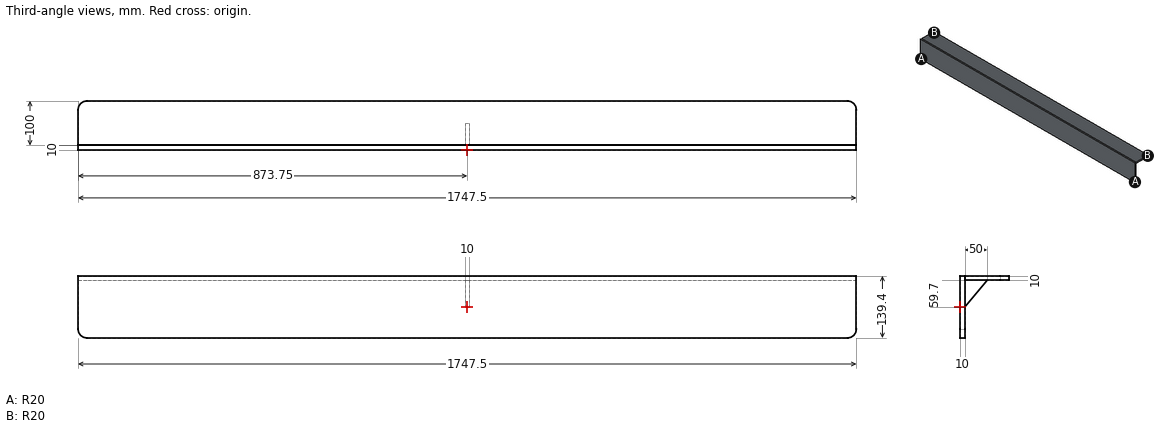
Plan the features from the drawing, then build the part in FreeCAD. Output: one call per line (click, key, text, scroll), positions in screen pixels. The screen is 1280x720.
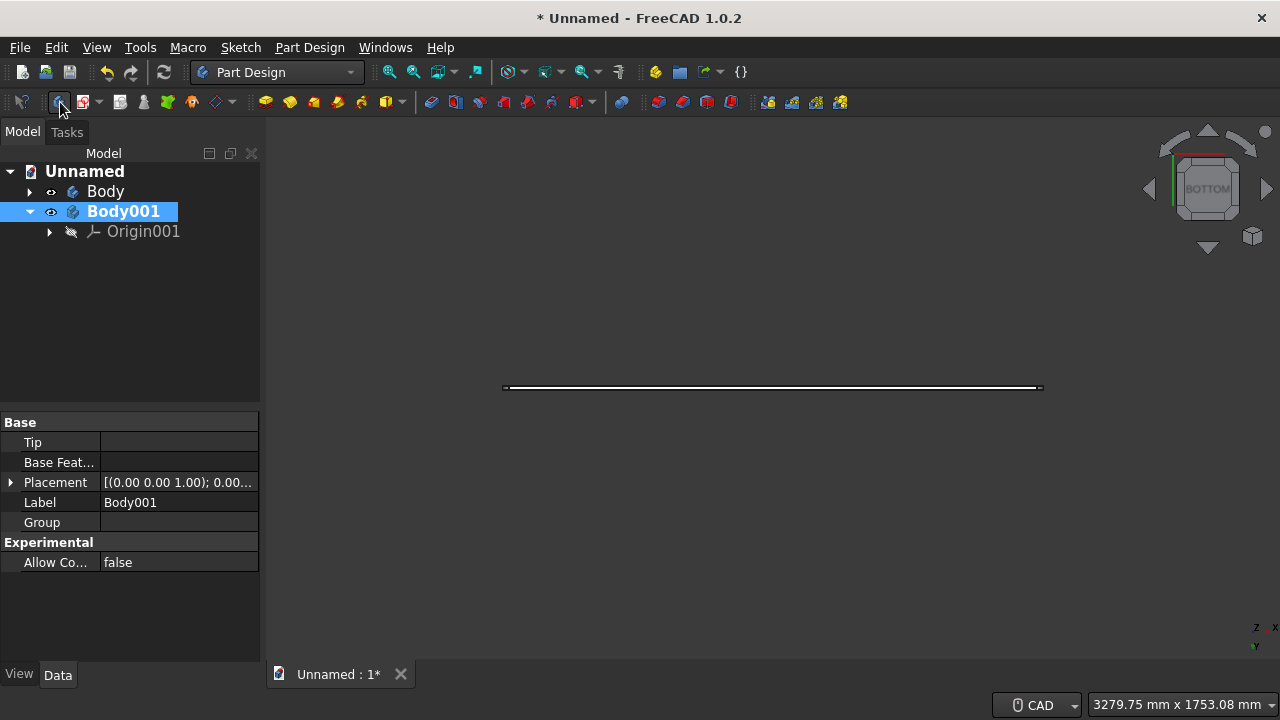
click(50, 232)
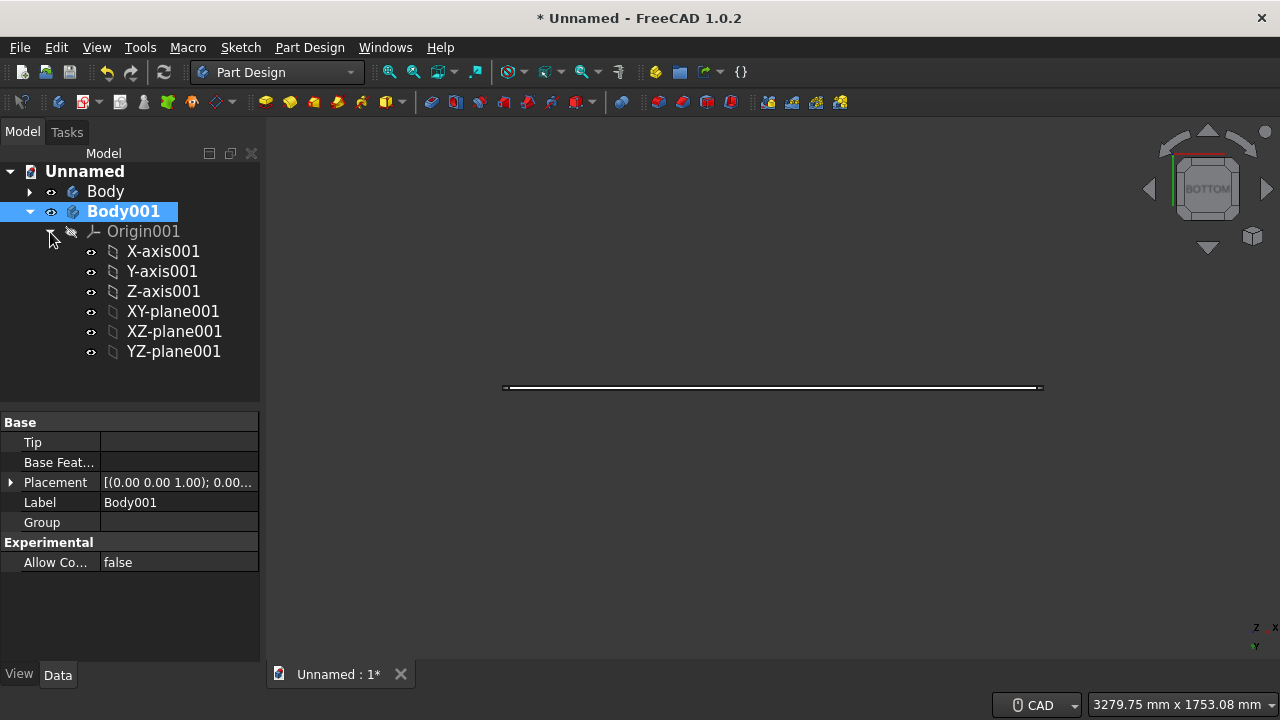
click(136, 312)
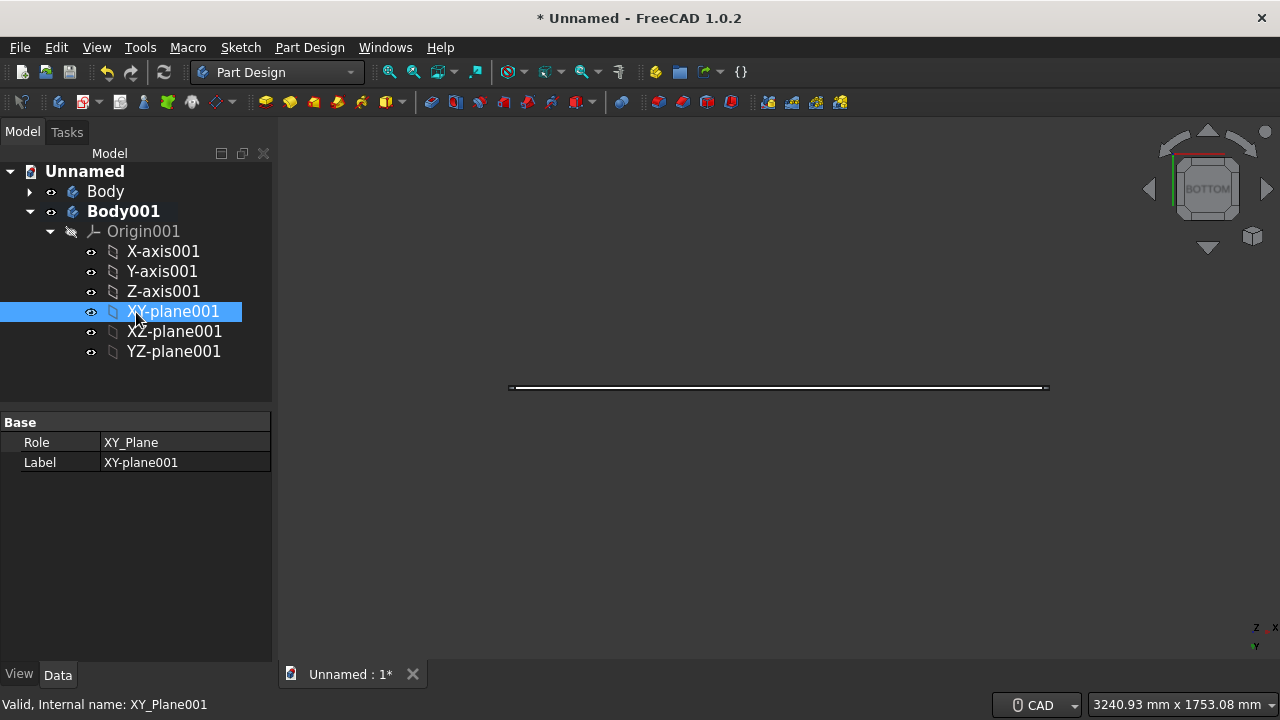
click(216, 102)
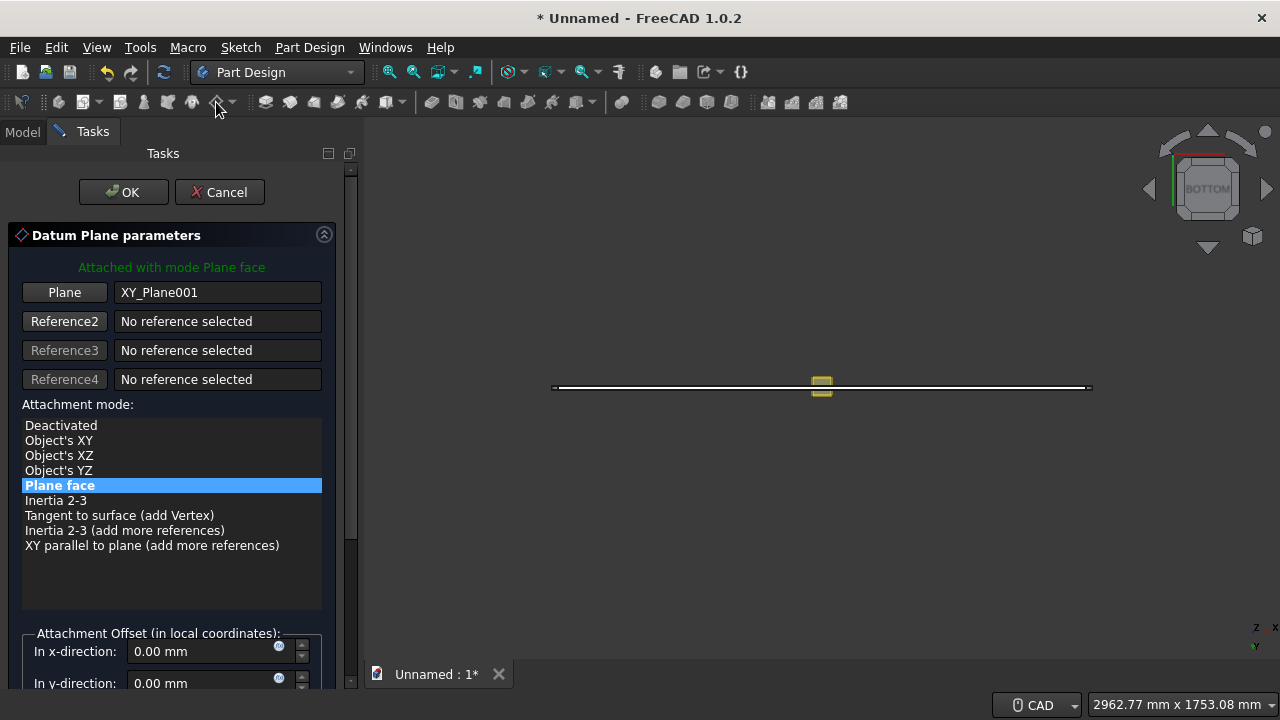
scroll(351, 426, down, 2)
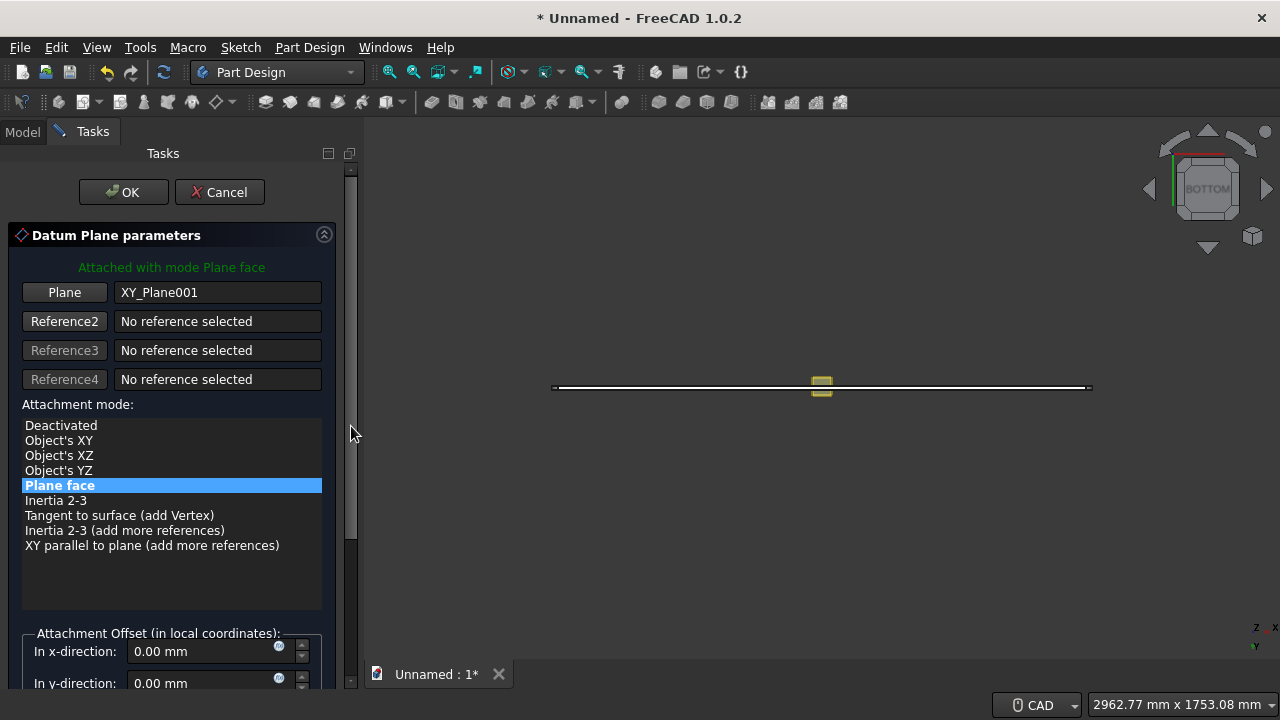
triple_click(210, 595)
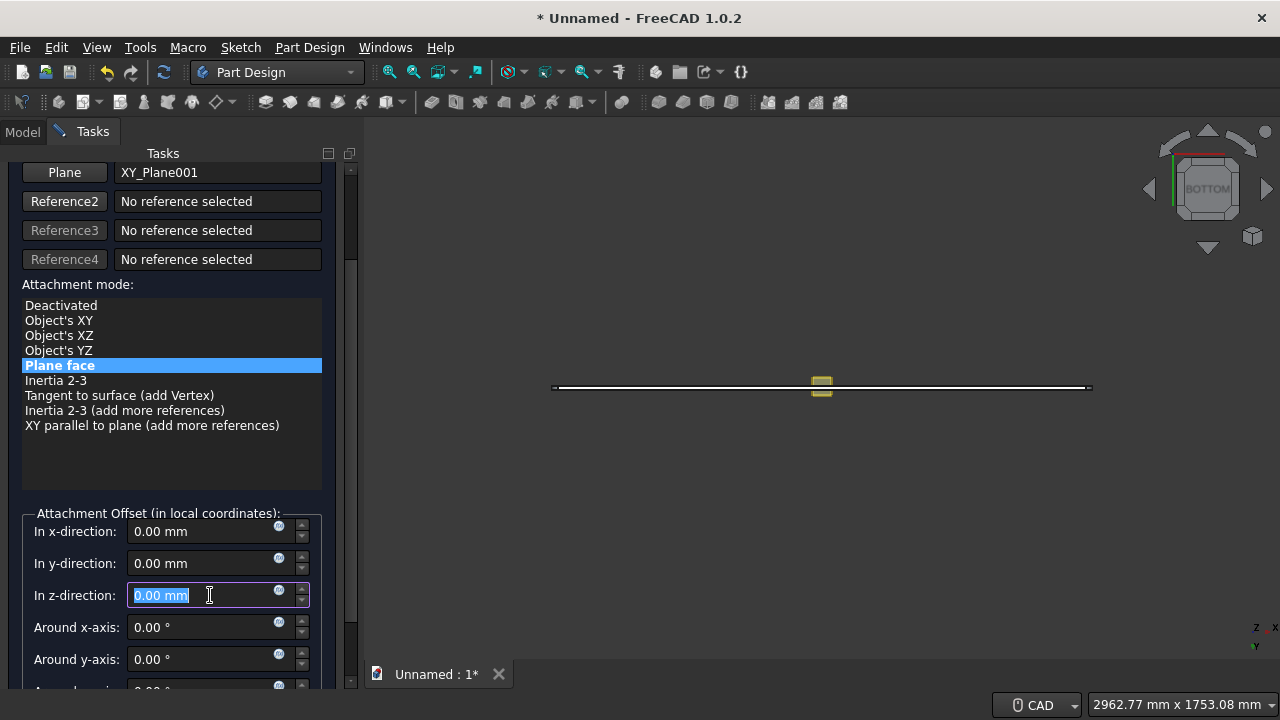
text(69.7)
key(Tab)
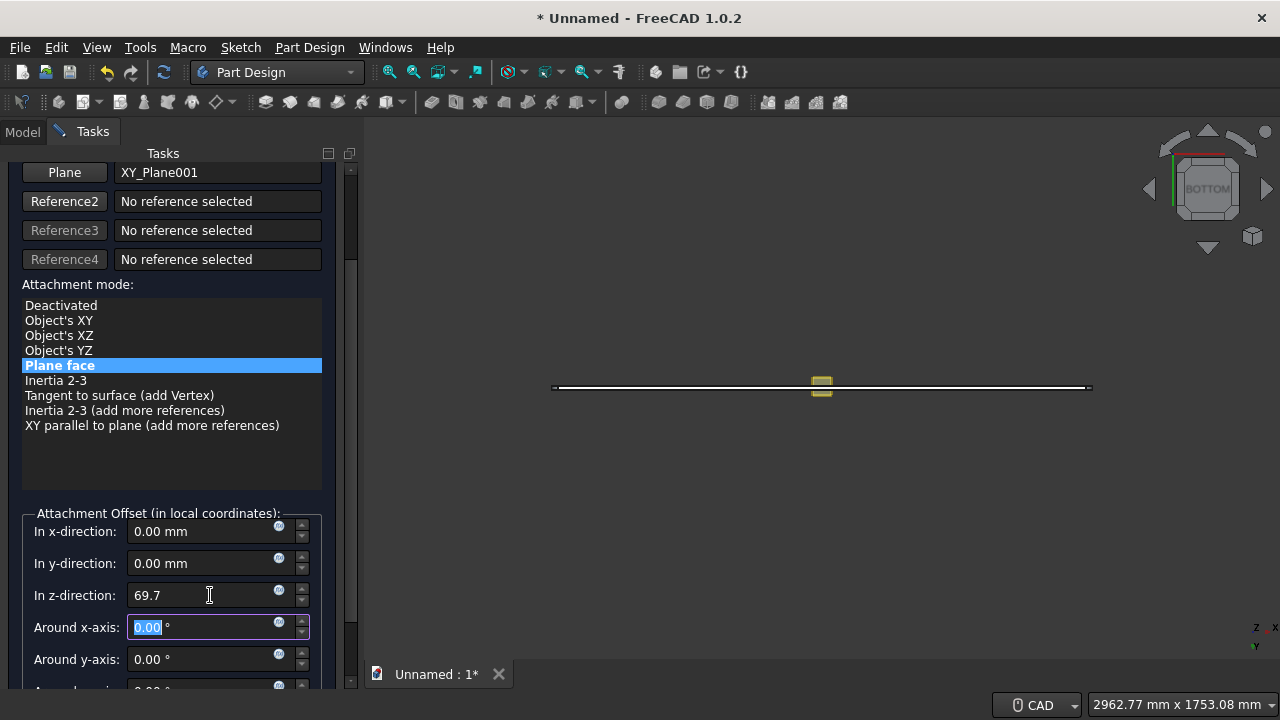
scroll(351, 426, up, 3)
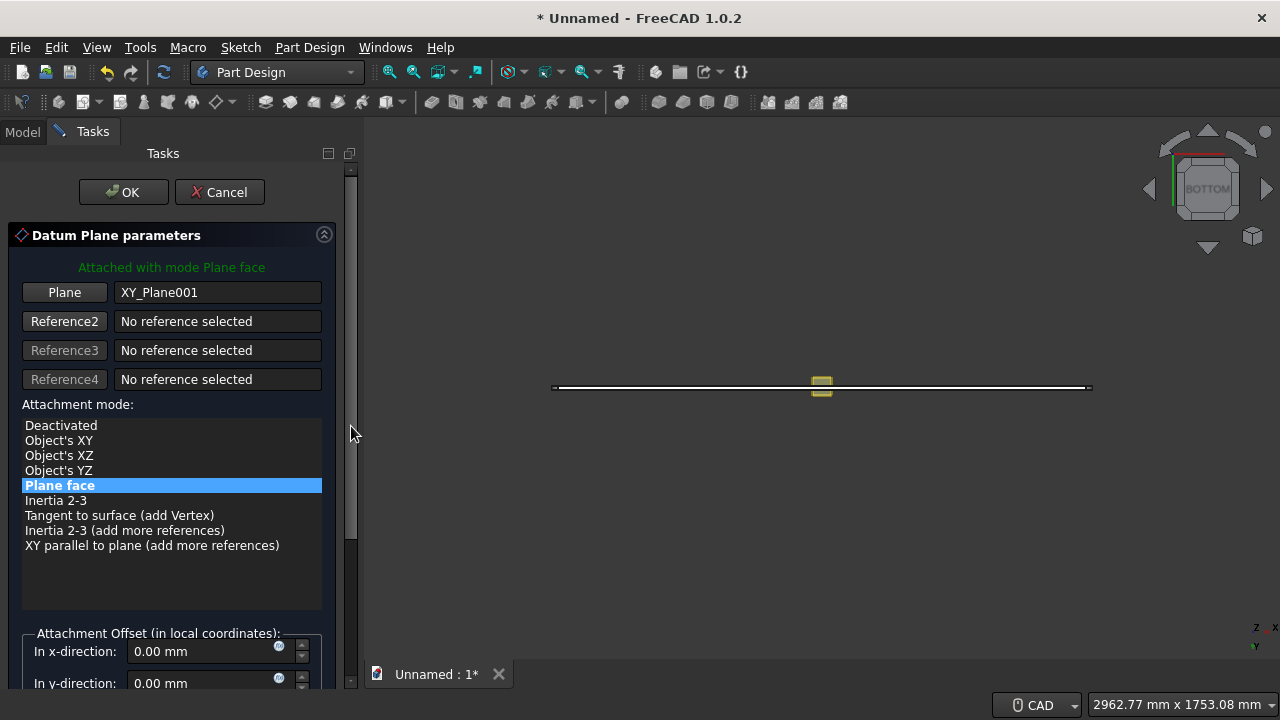
click(124, 192)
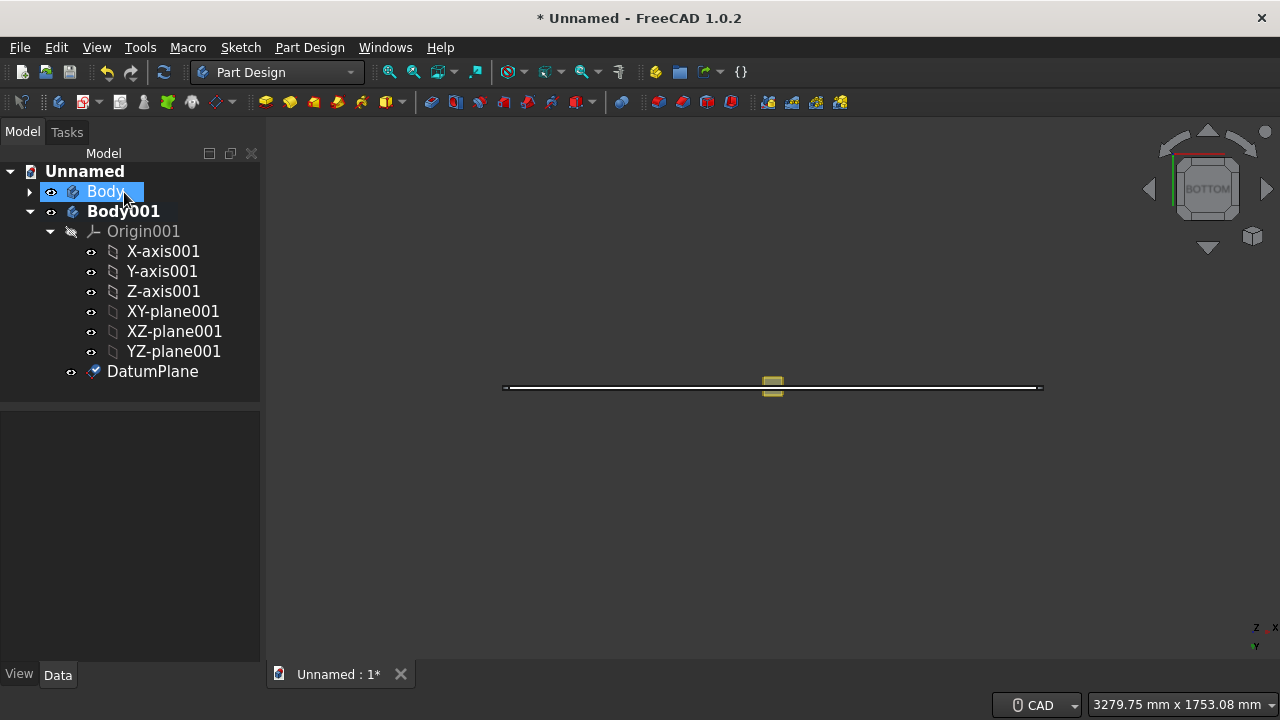
click(116, 372)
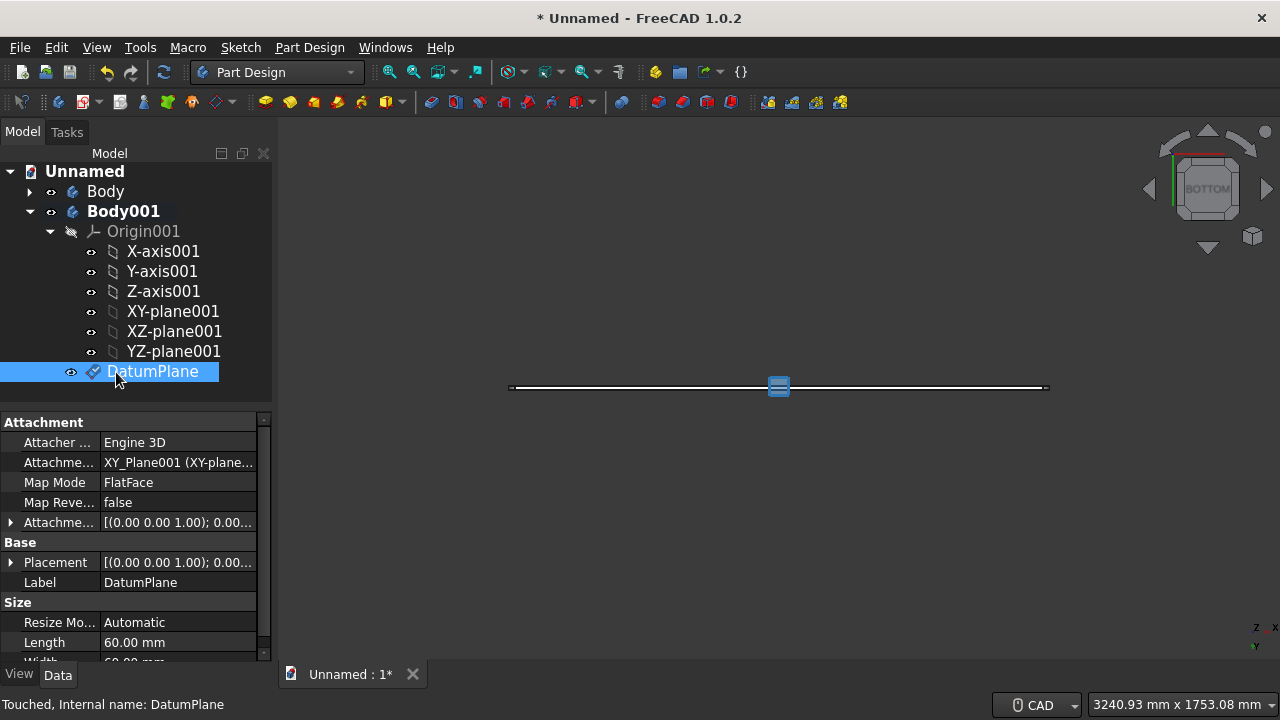
click(84, 102)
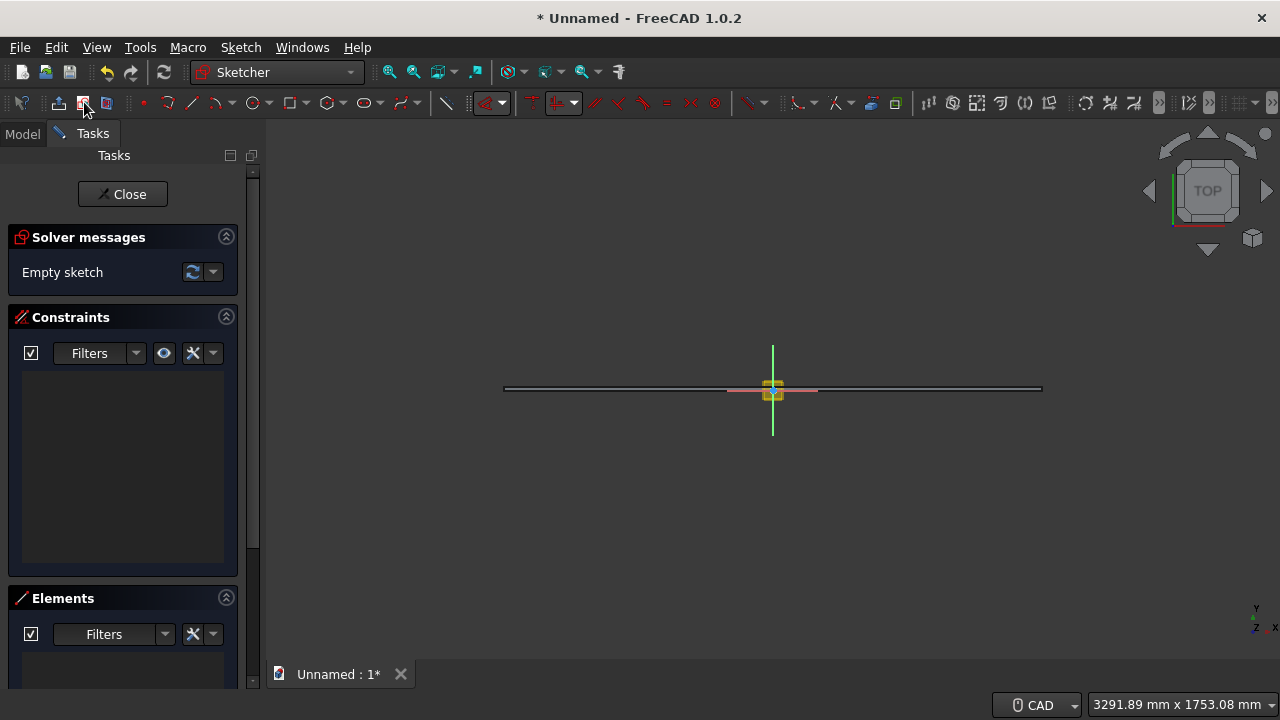
click(290, 104)